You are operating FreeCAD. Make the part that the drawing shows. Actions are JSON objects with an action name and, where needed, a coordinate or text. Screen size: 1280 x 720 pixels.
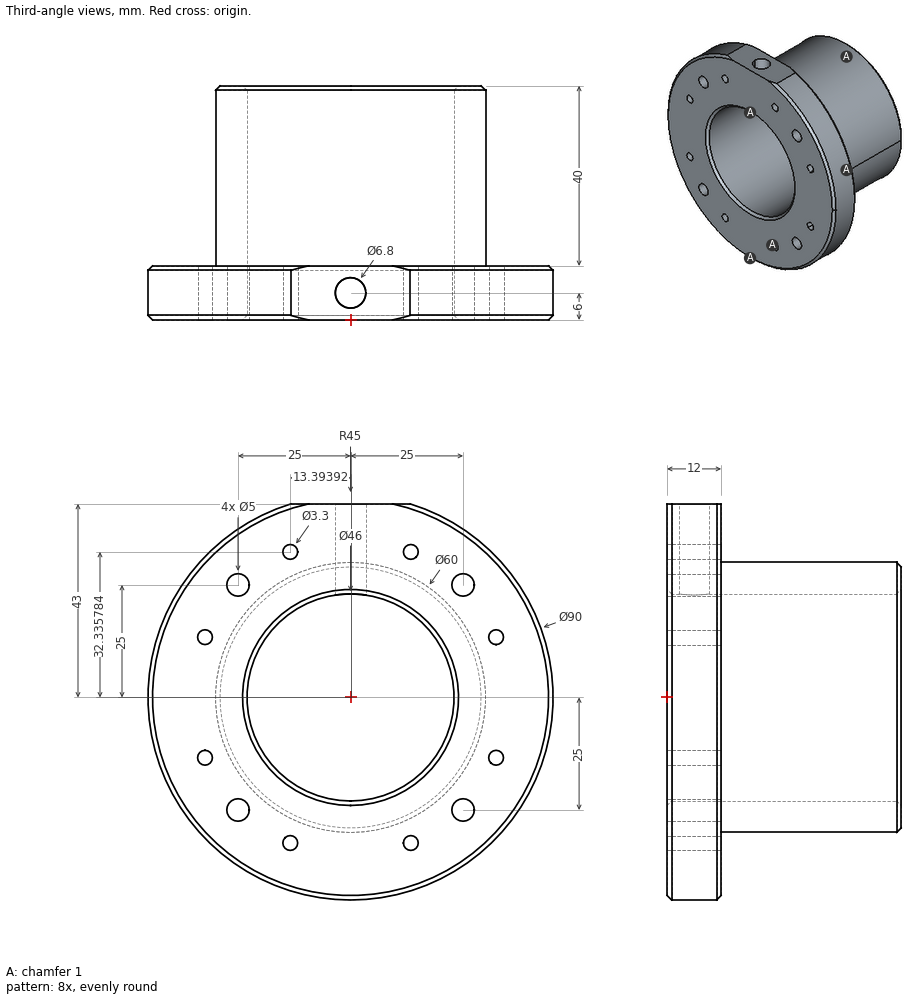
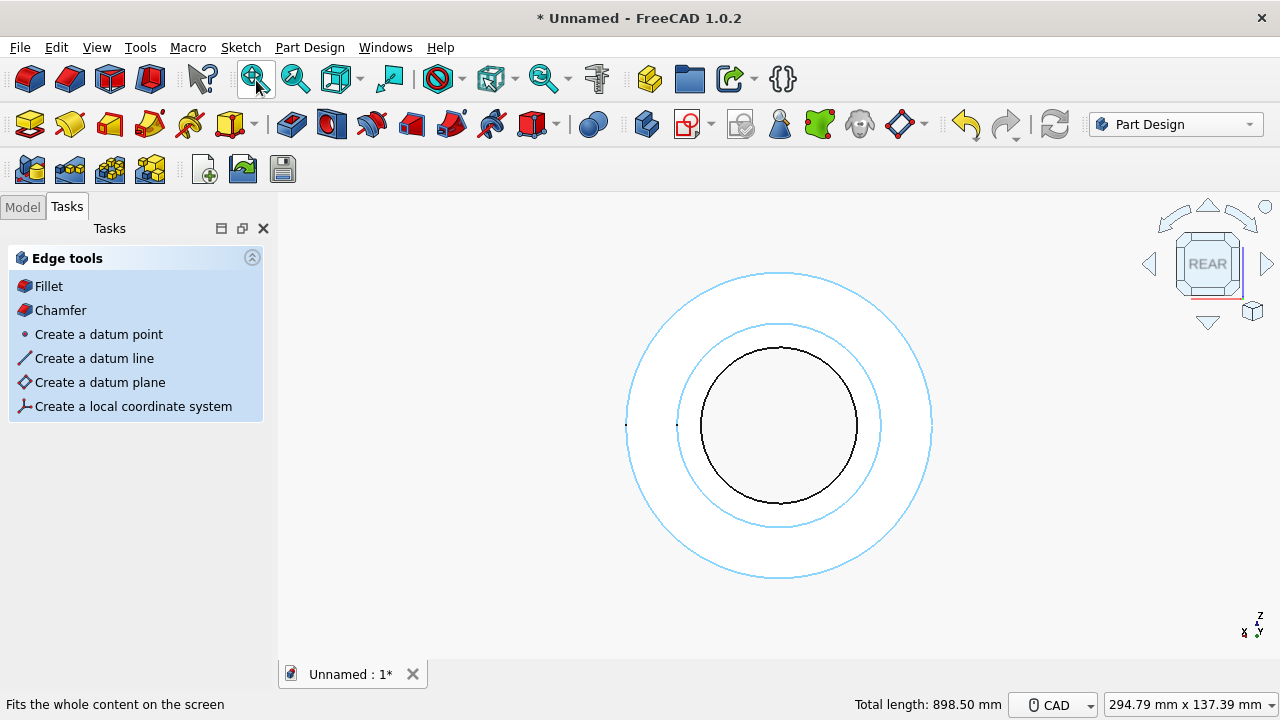
{"action": "left_click", "coordinate": [857, 424], "text": "ctrl"}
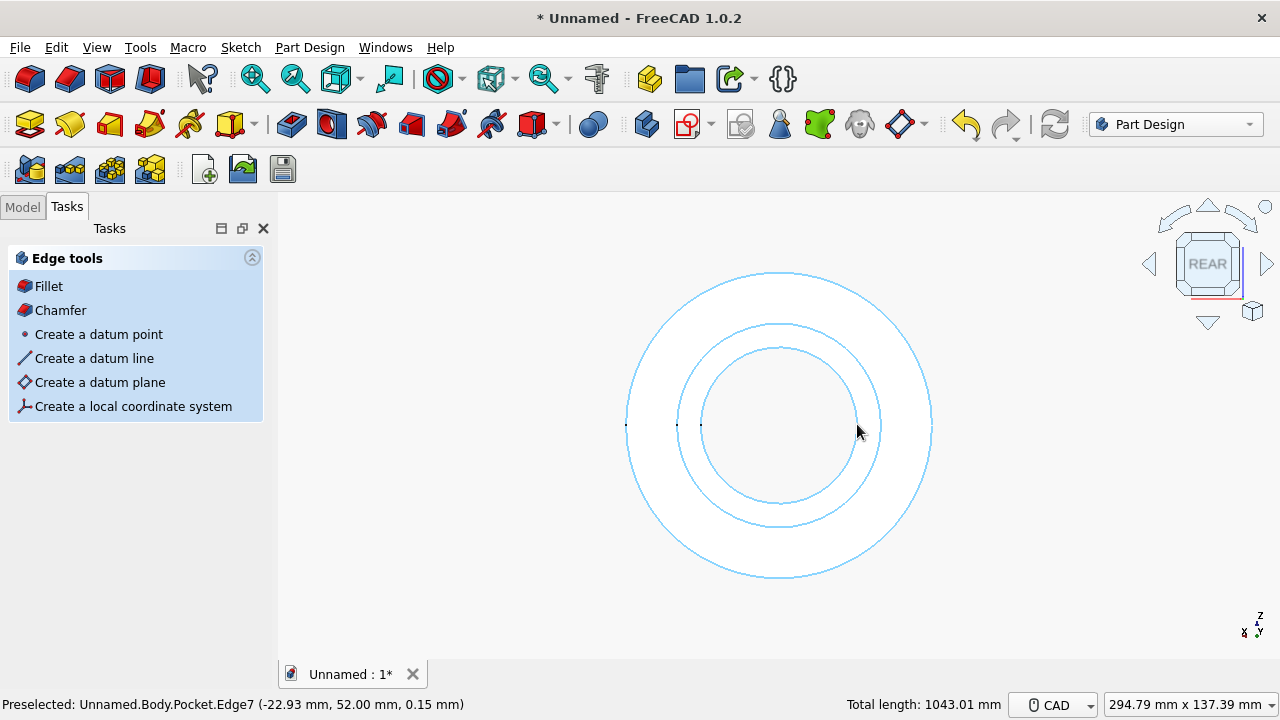
{"action": "left_click", "coordinate": [70, 80]}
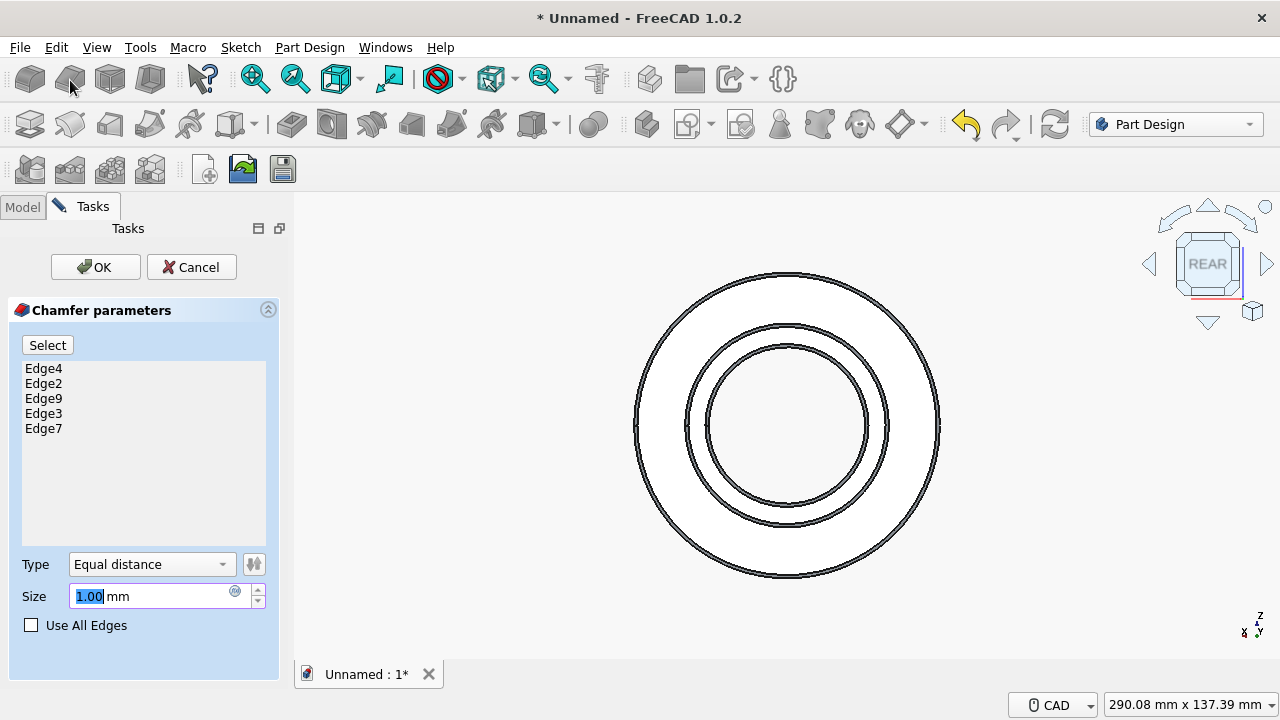
{"action": "type", "text": "1"}
{"action": "key", "text": "Tab"}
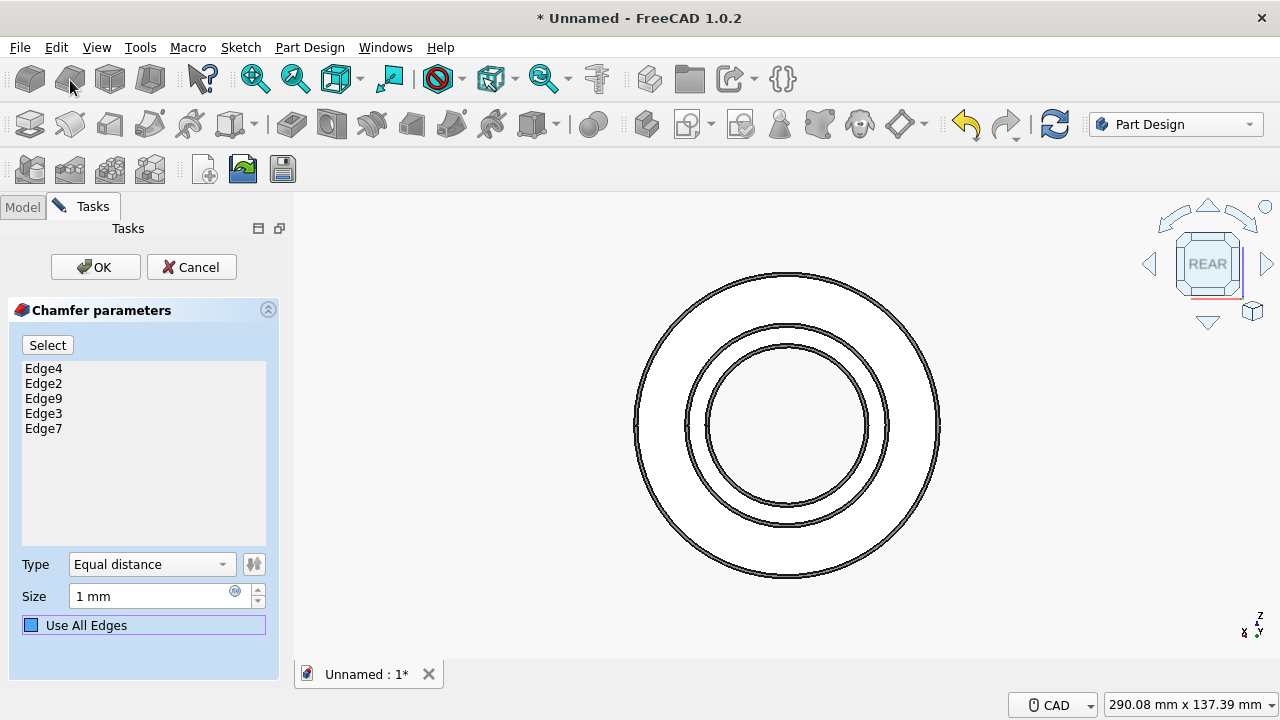
{"action": "left_click", "coordinate": [96, 267]}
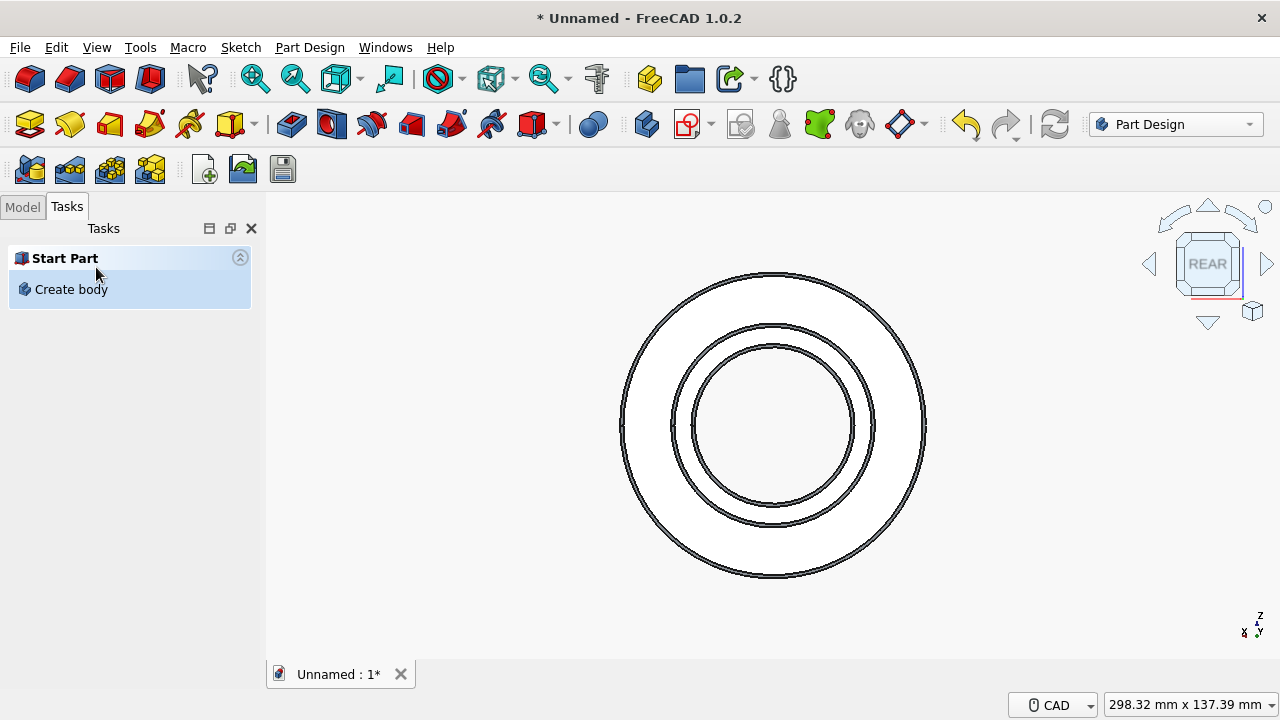
{"action": "left_click", "coordinate": [688, 124]}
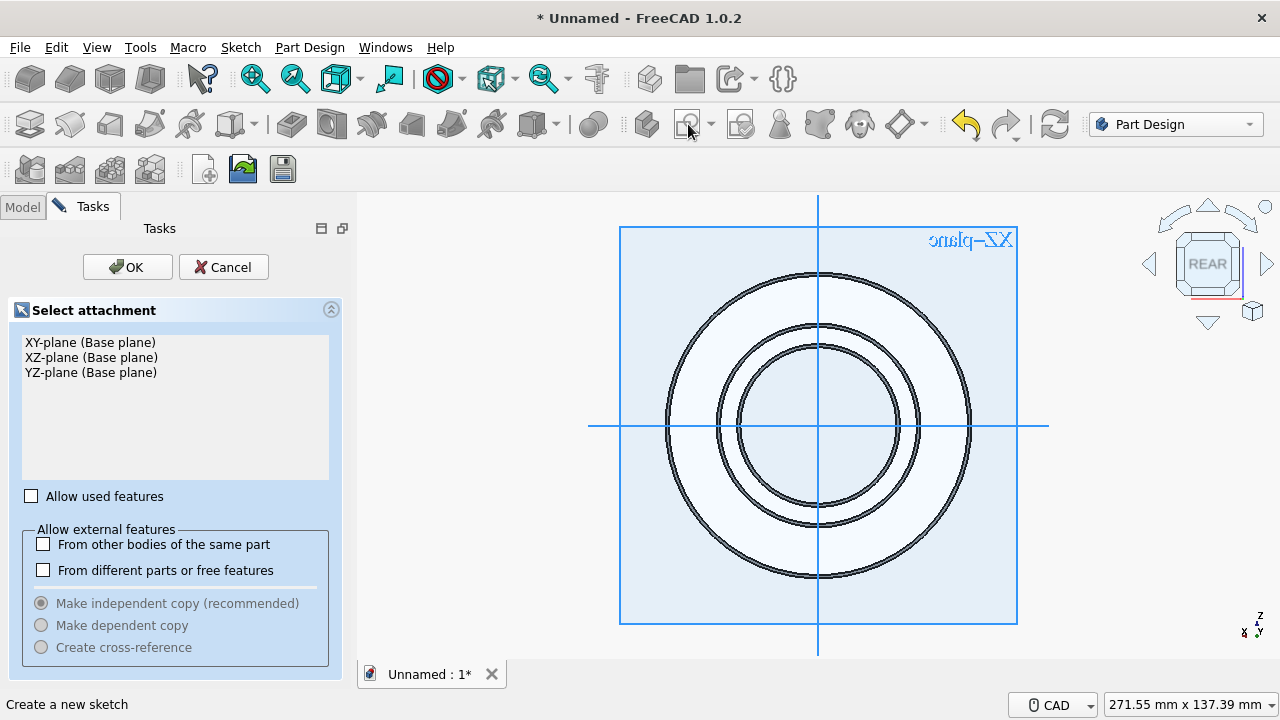
{"action": "left_click", "coordinate": [82, 358]}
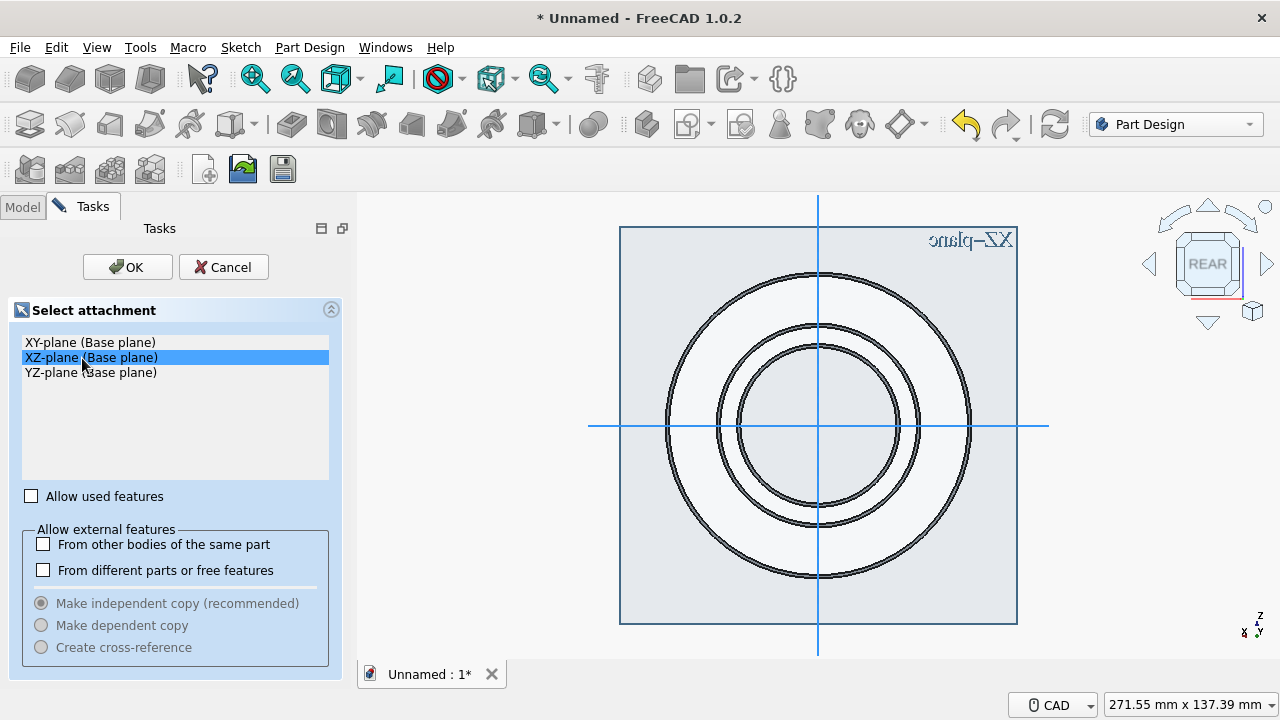
{"action": "left_click", "coordinate": [128, 267]}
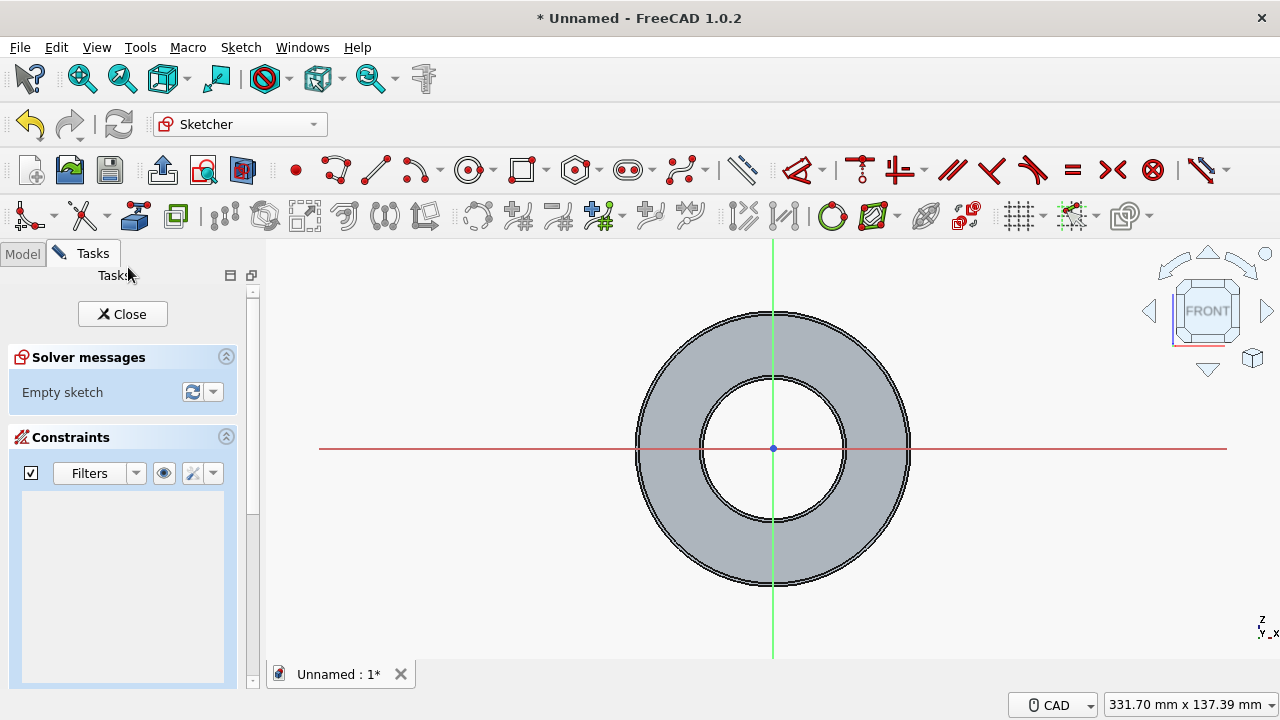
{"action": "scroll", "coordinate": [912, 449], "scroll_direction": "up", "scroll_amount": 2}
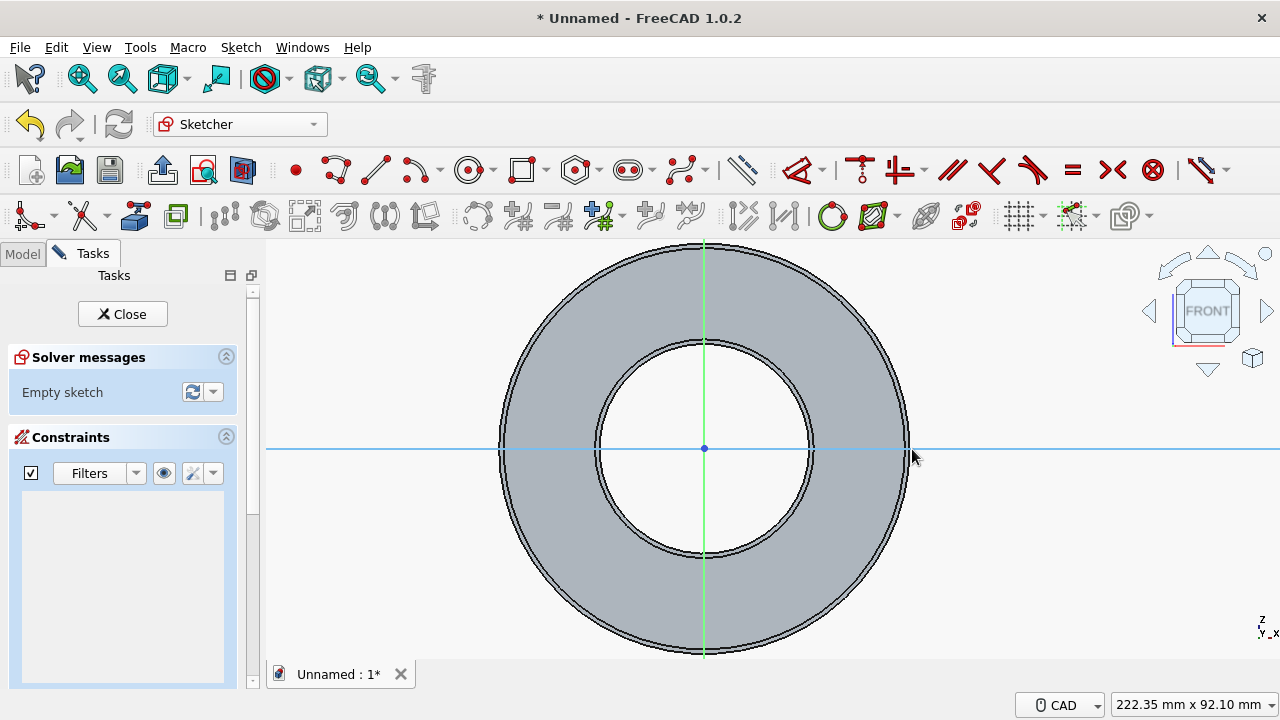
{"action": "key", "text": "g c"}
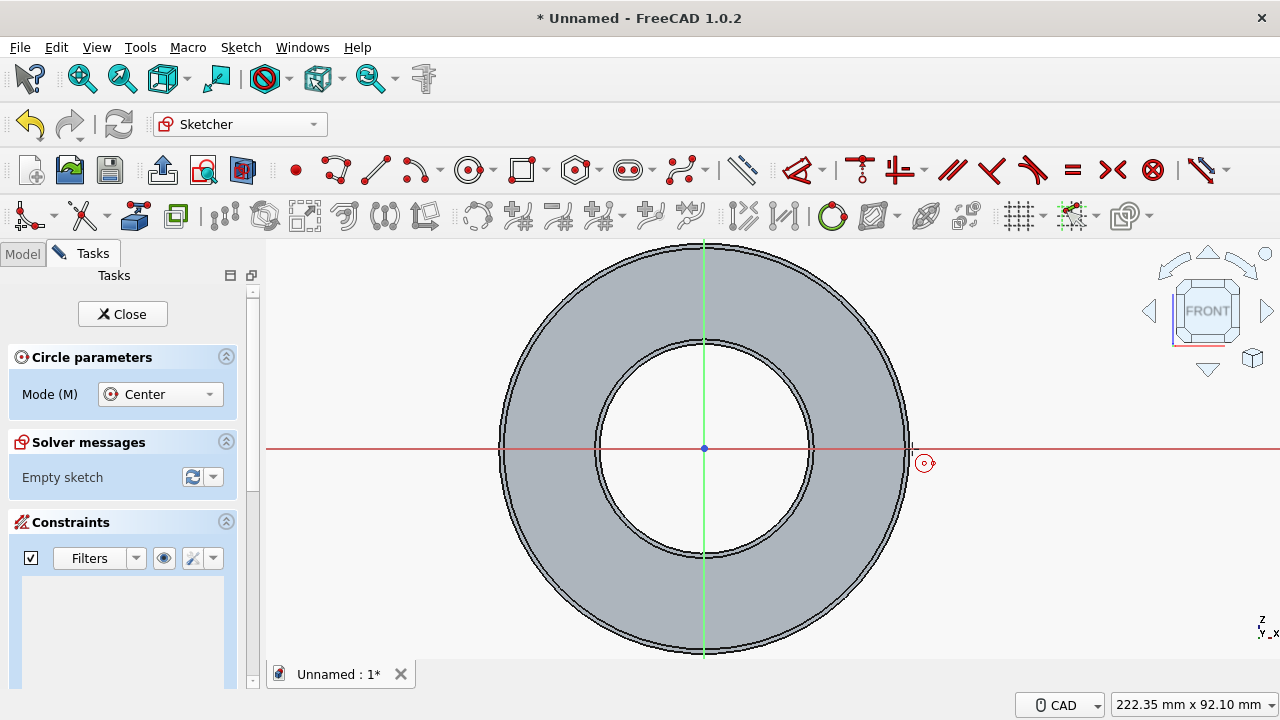
{"action": "scroll", "coordinate": [590, 335], "scroll_direction": "up", "scroll_amount": 4}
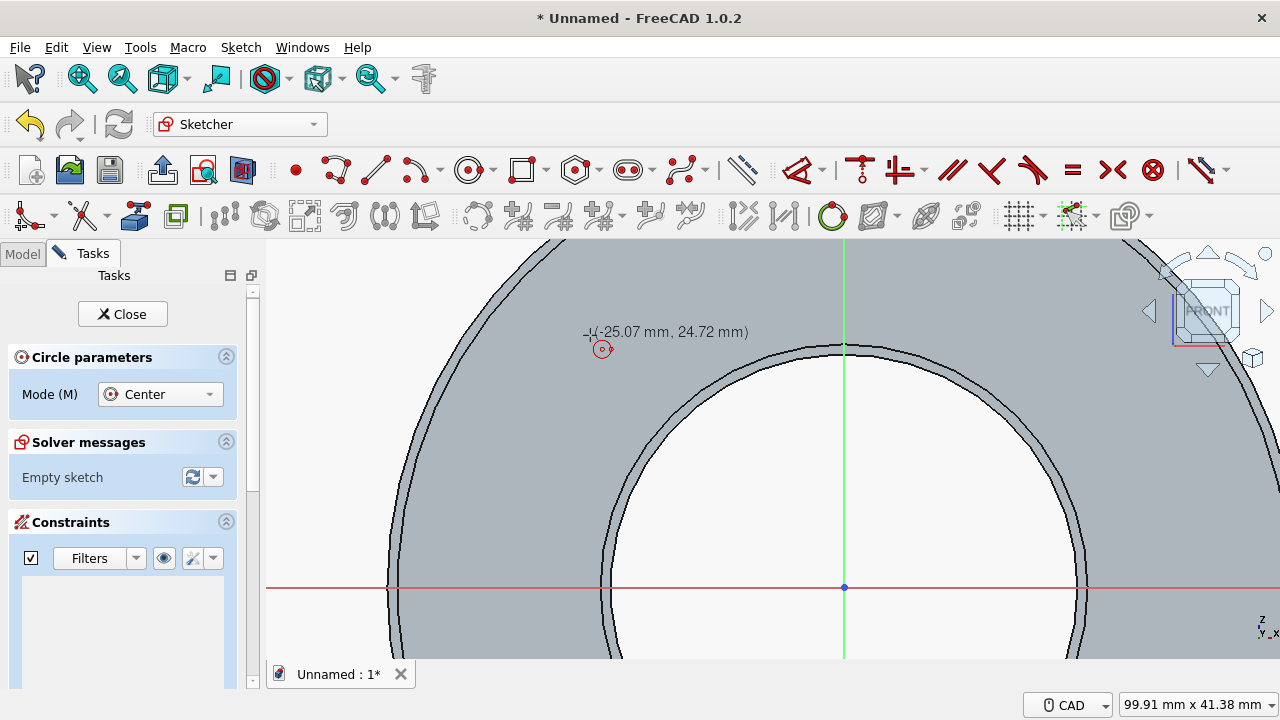
{"action": "left_click", "coordinate": [590, 334]}
{"action": "left_click", "coordinate": [608, 316]}